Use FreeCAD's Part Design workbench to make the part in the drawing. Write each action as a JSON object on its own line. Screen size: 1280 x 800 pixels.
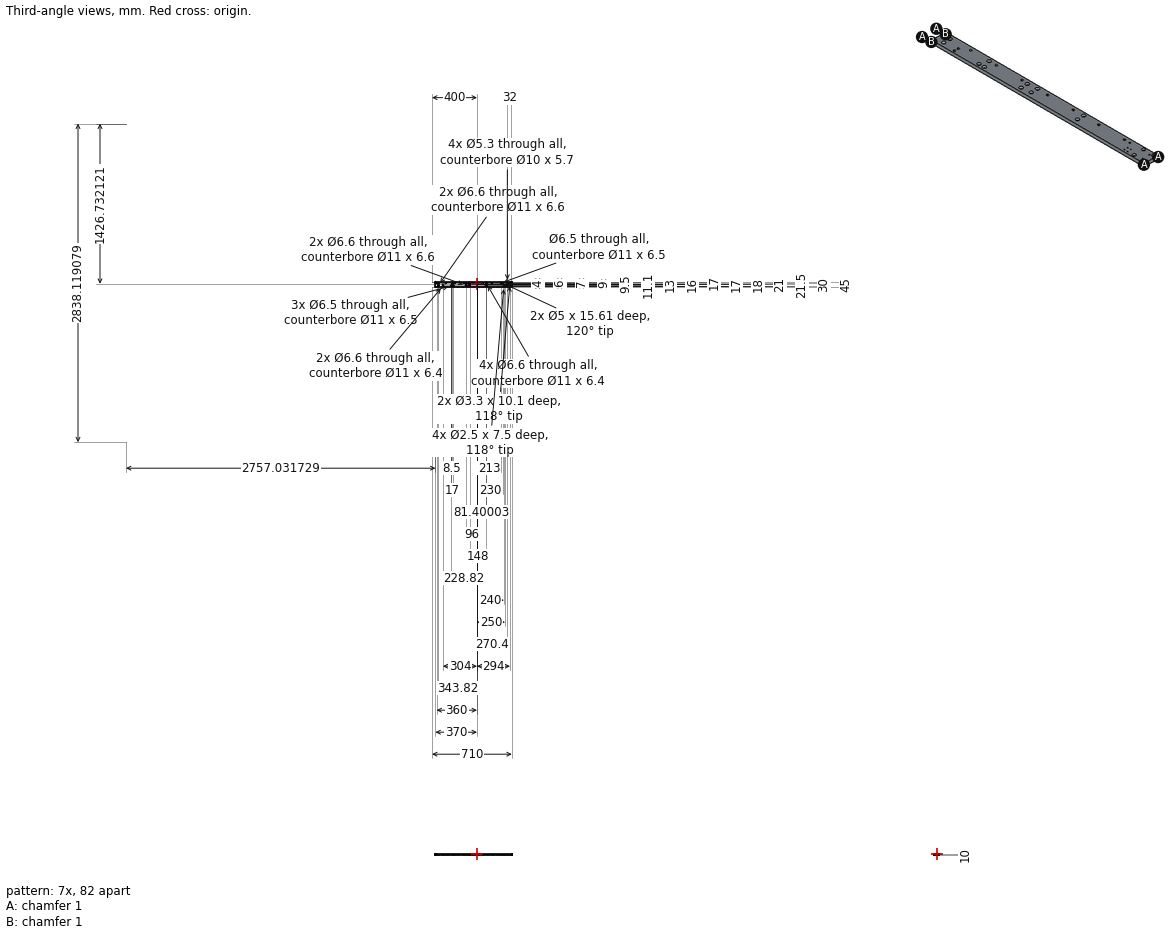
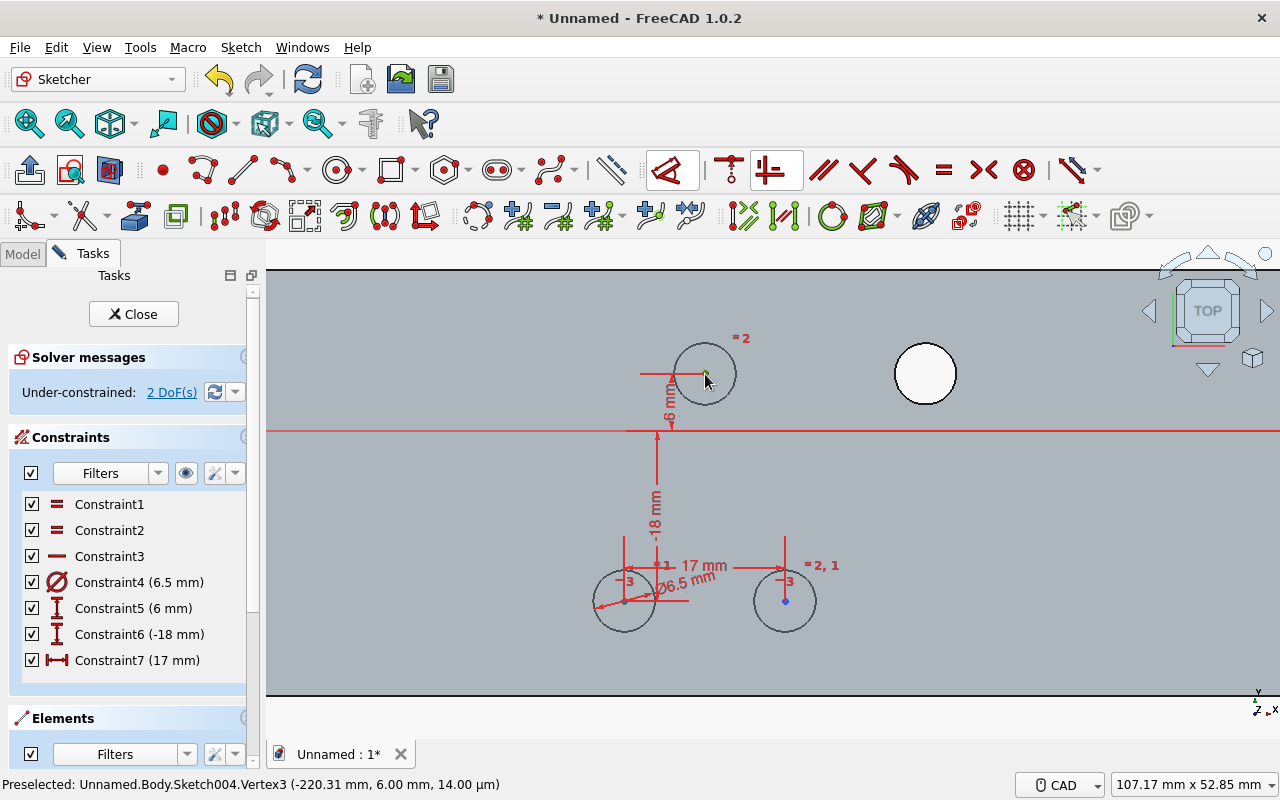
{"action": "key", "text": "l"}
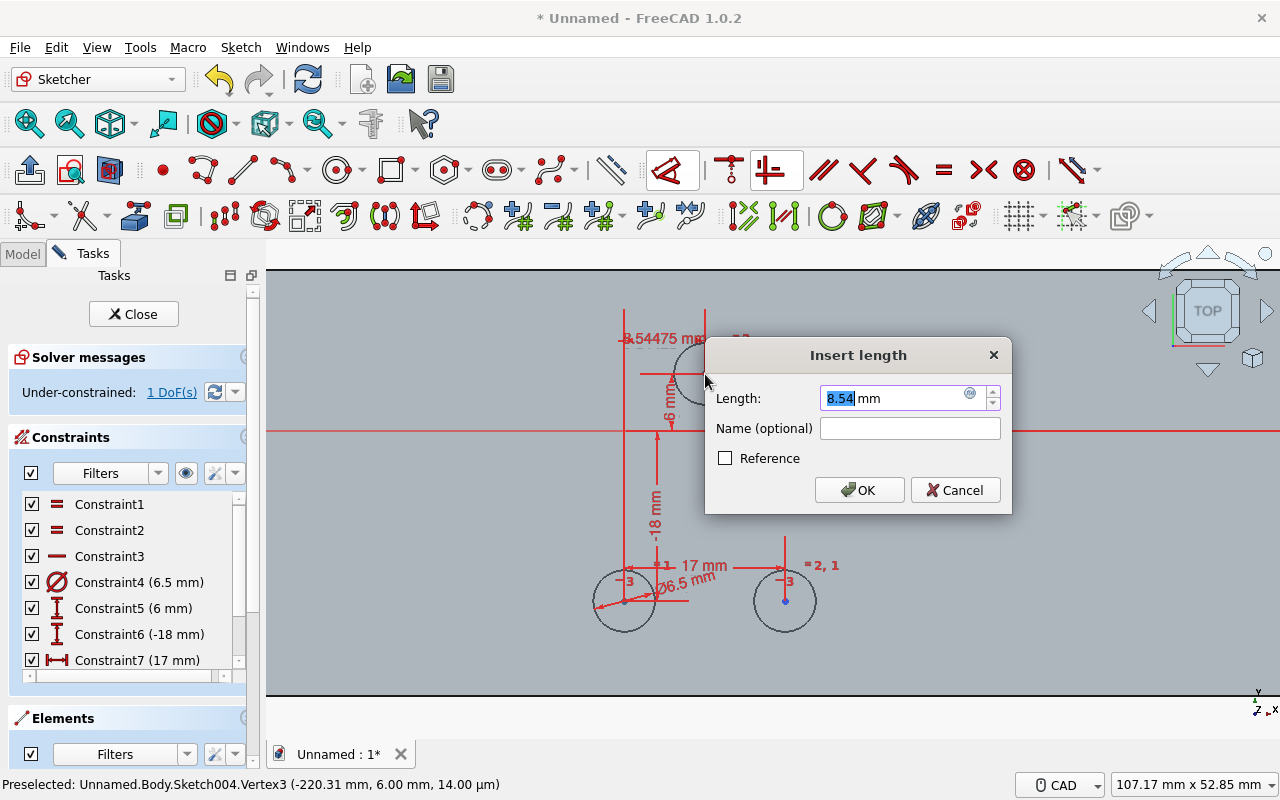
{"action": "type", "text": "8.5"}
{"action": "key", "text": "Return"}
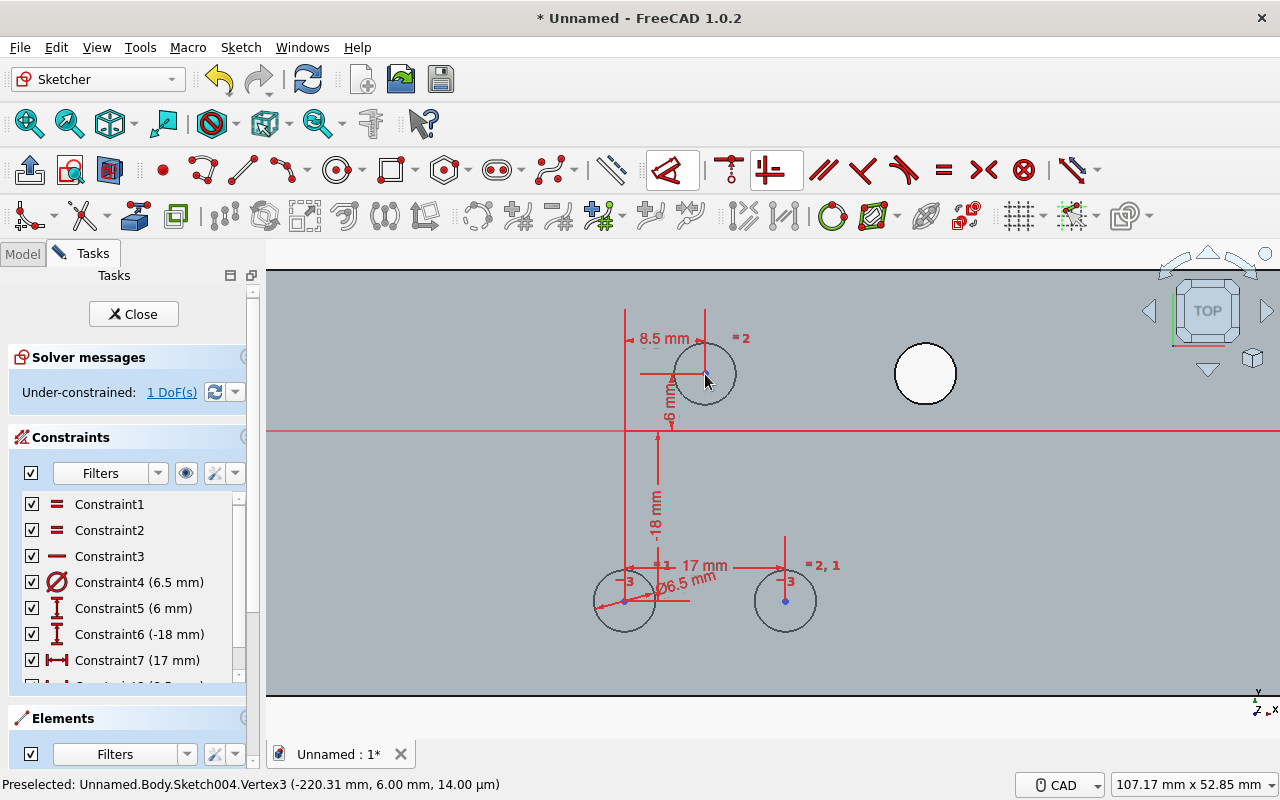
{"action": "left_click", "coordinate": [625, 601]}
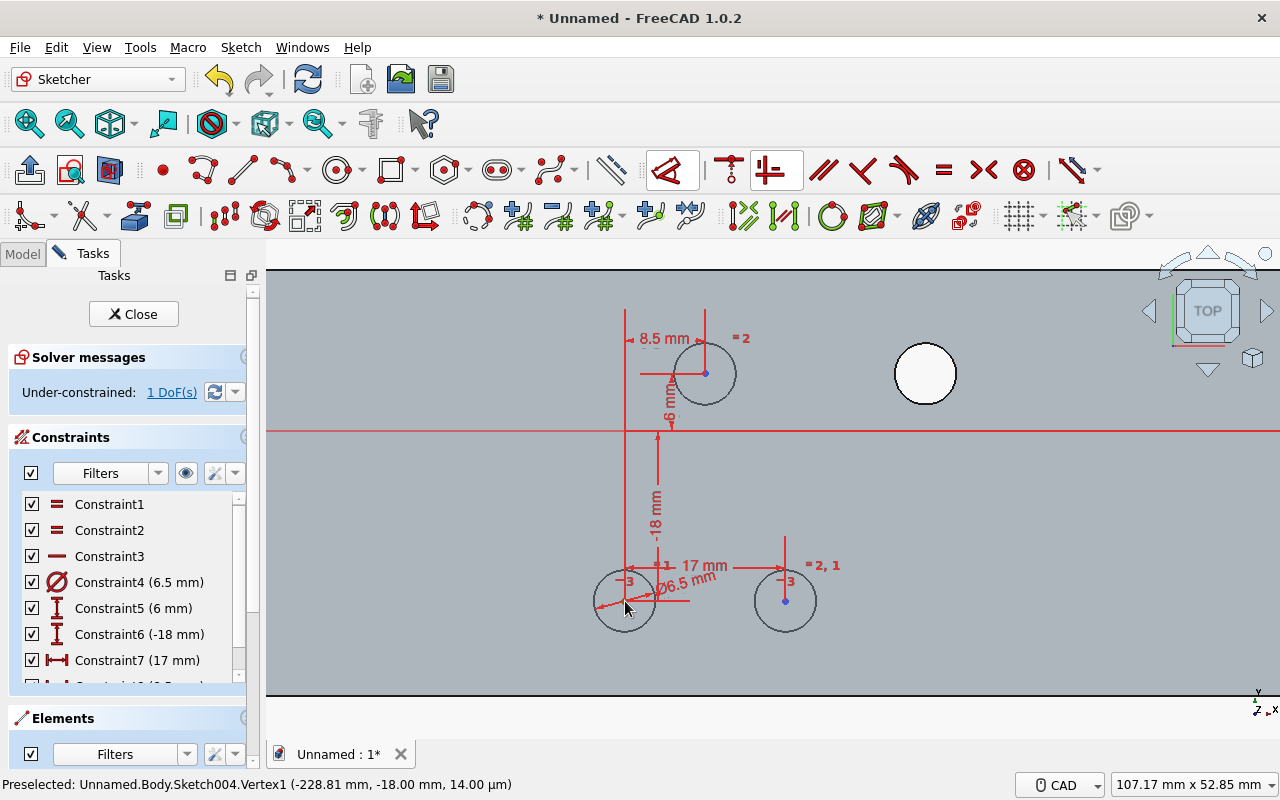
{"action": "left_click", "coordinate": [694, 170]}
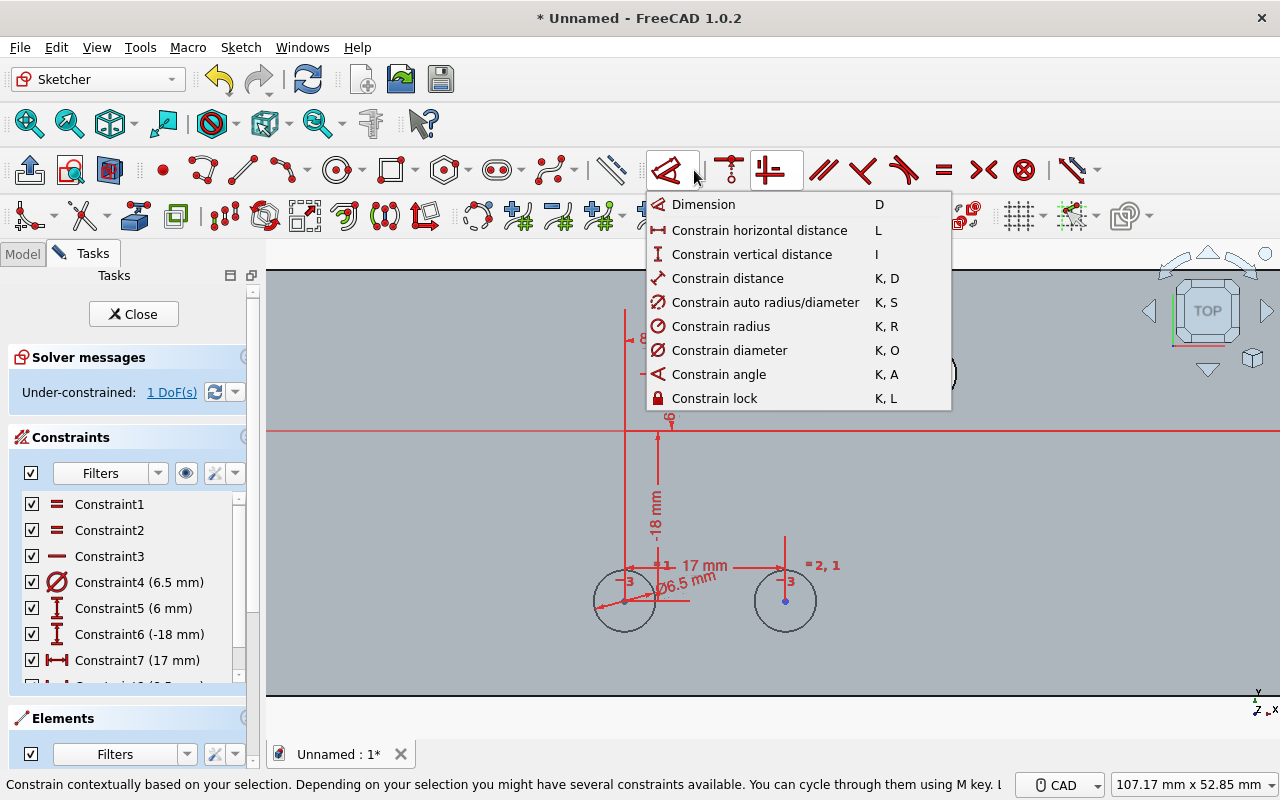
{"action": "left_click", "coordinate": [799, 230]}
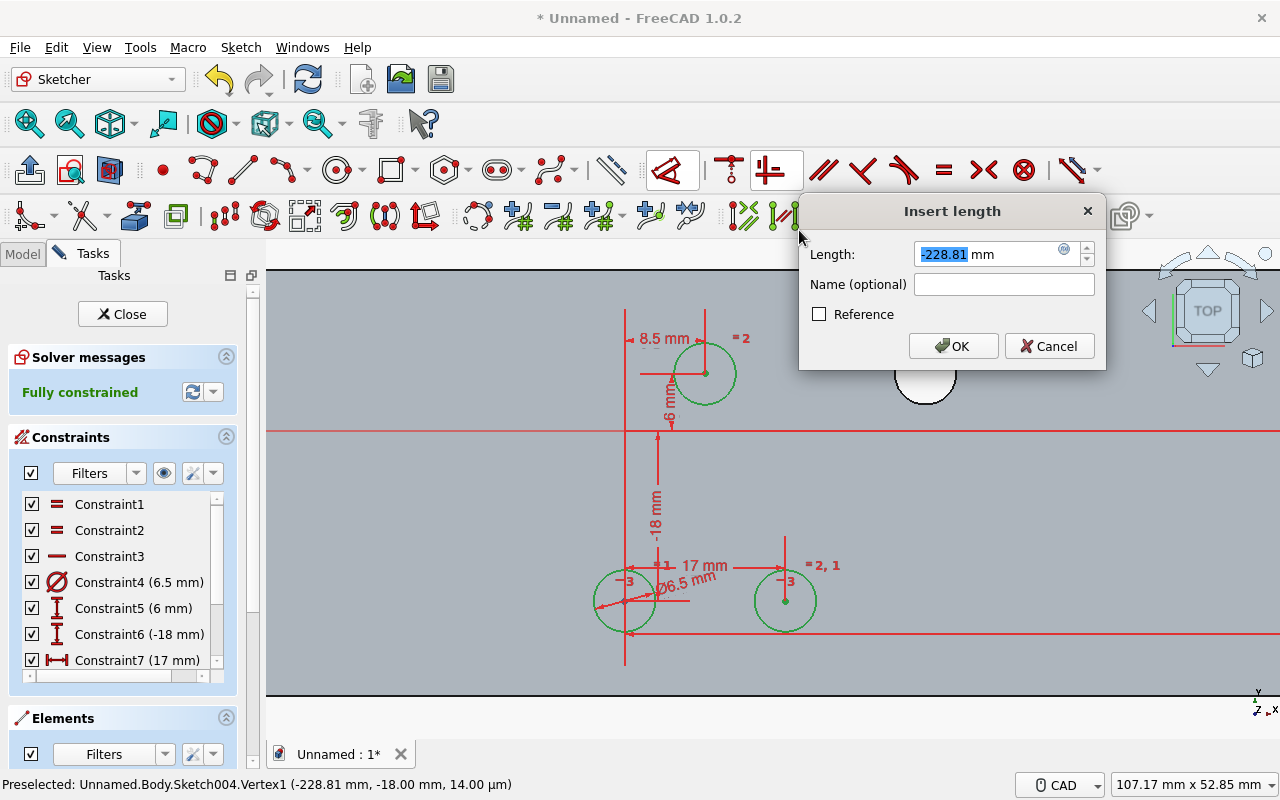
{"action": "type", "text": "-228.82"}
{"action": "key", "text": "Return"}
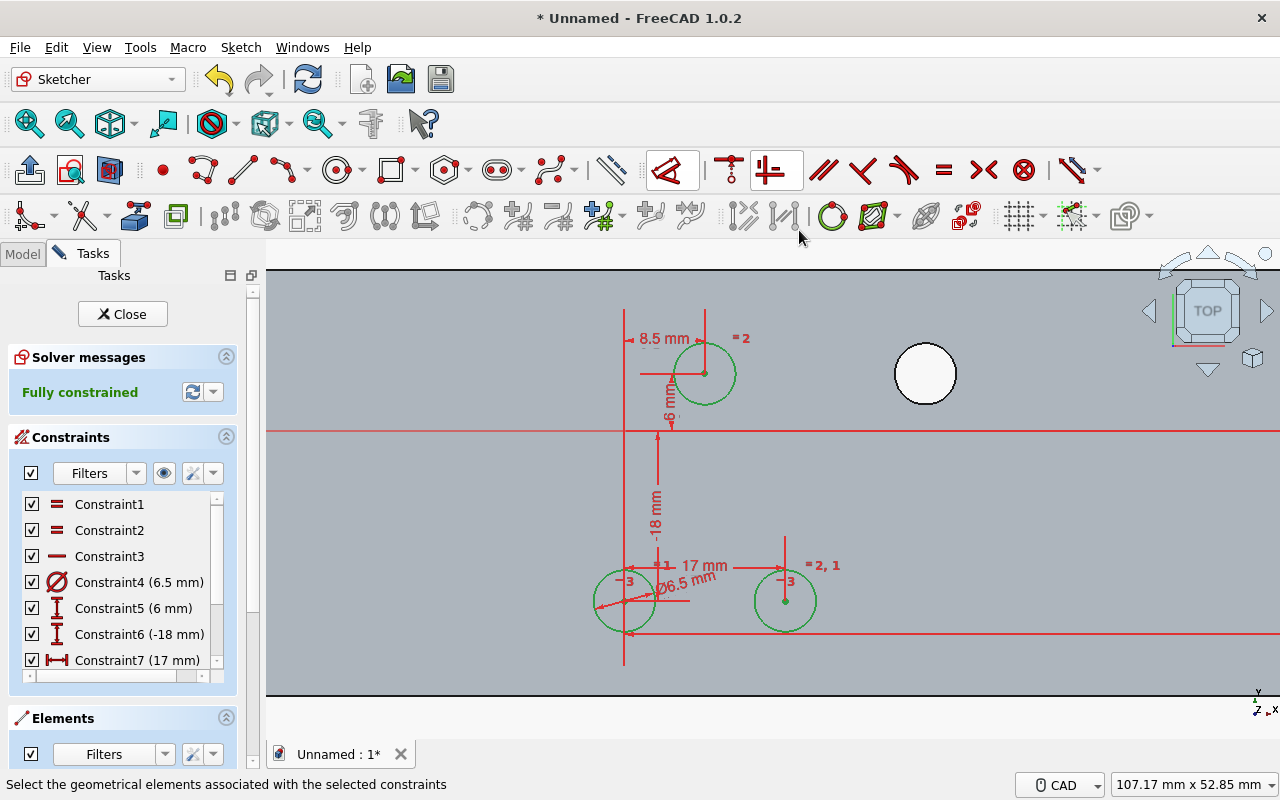
{"action": "left_click", "coordinate": [123, 314]}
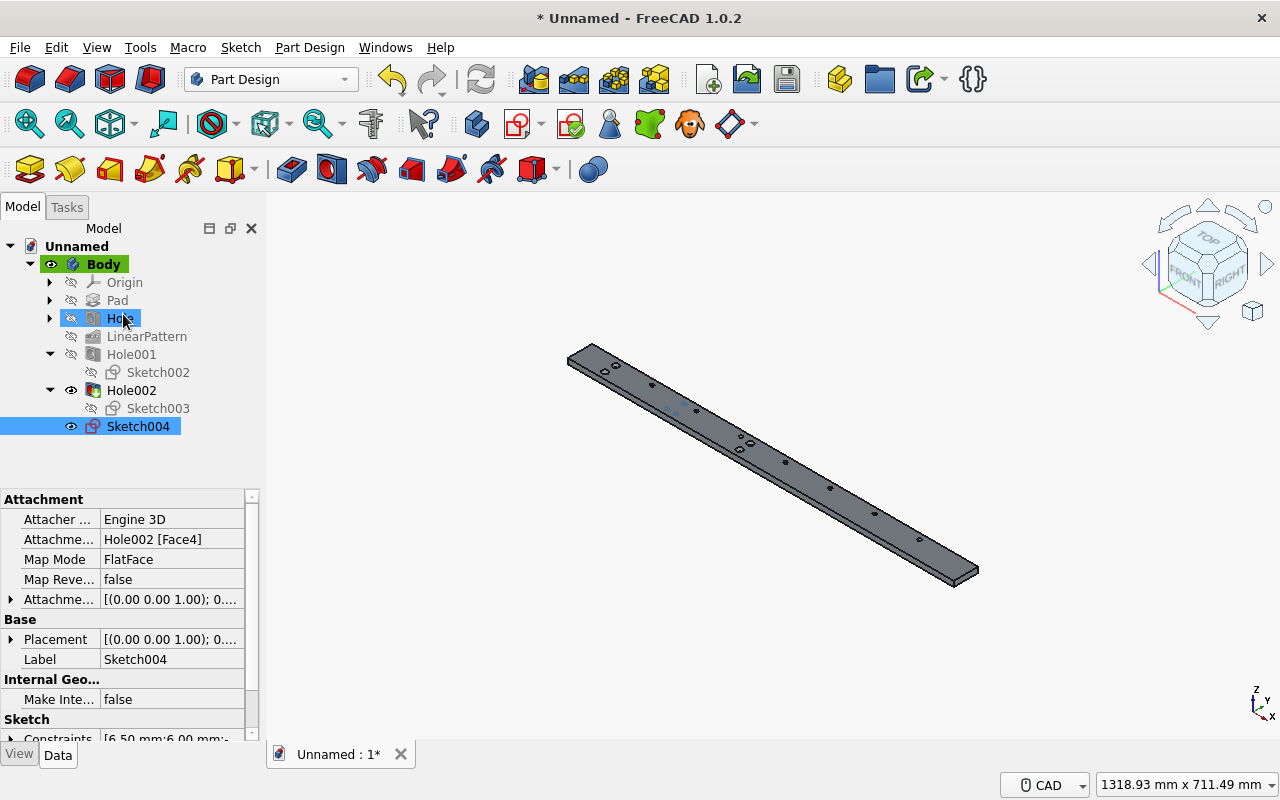
{"action": "left_click", "coordinate": [332, 170]}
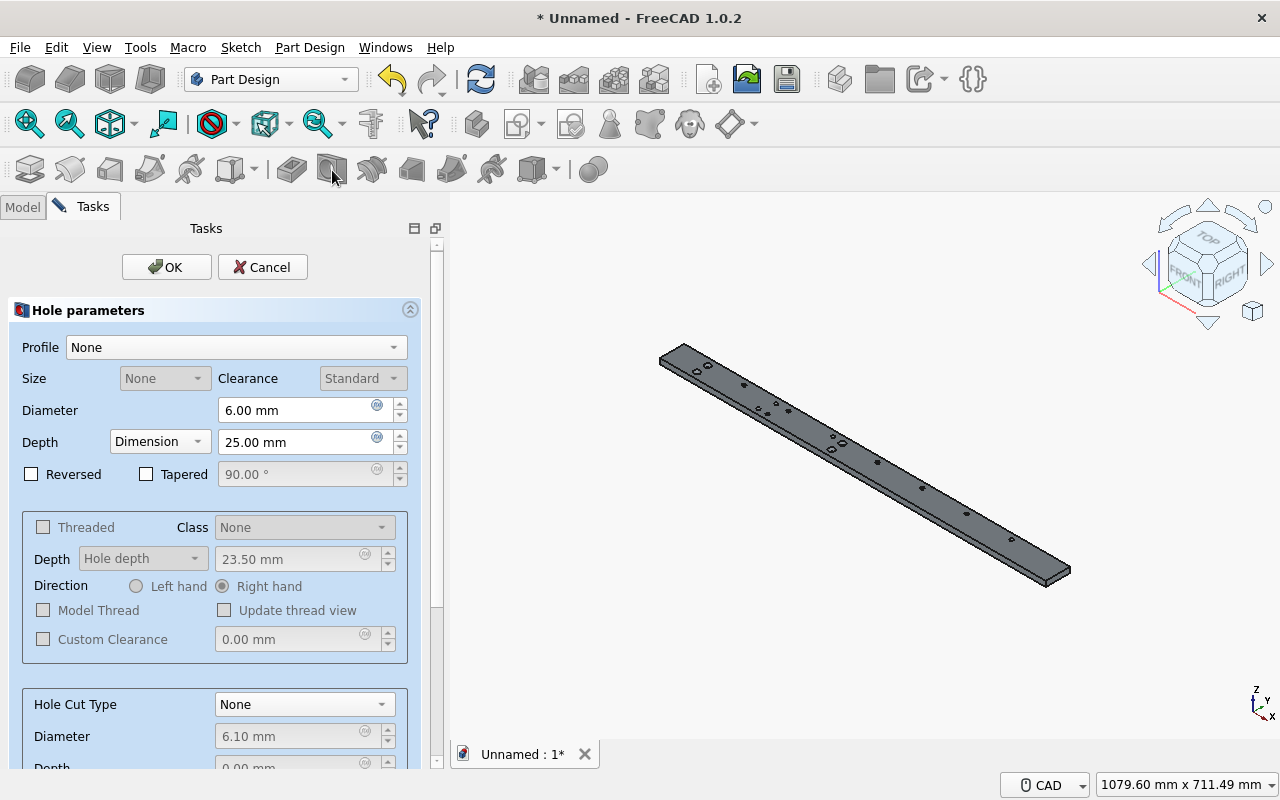
{"action": "triple_click", "coordinate": [305, 410]}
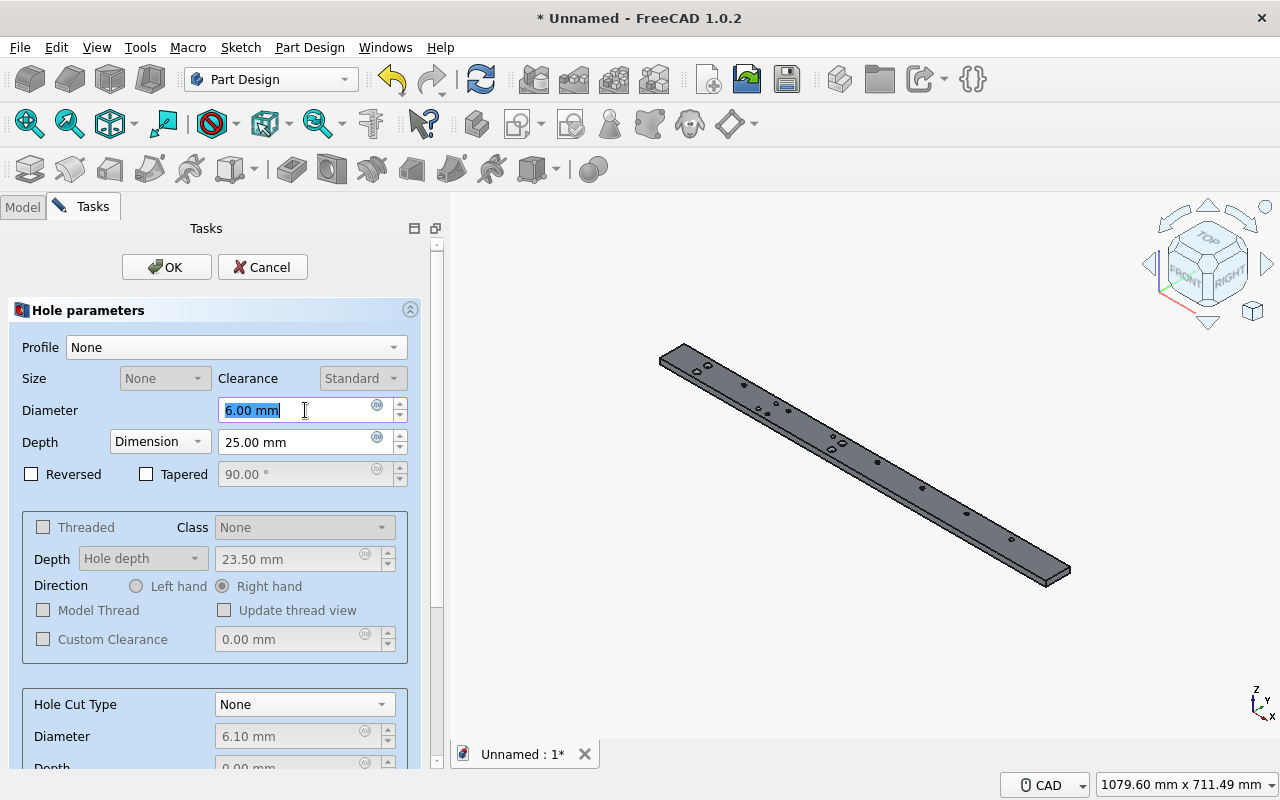
{"action": "type", "text": "6.5"}
{"action": "key", "text": "Tab"}